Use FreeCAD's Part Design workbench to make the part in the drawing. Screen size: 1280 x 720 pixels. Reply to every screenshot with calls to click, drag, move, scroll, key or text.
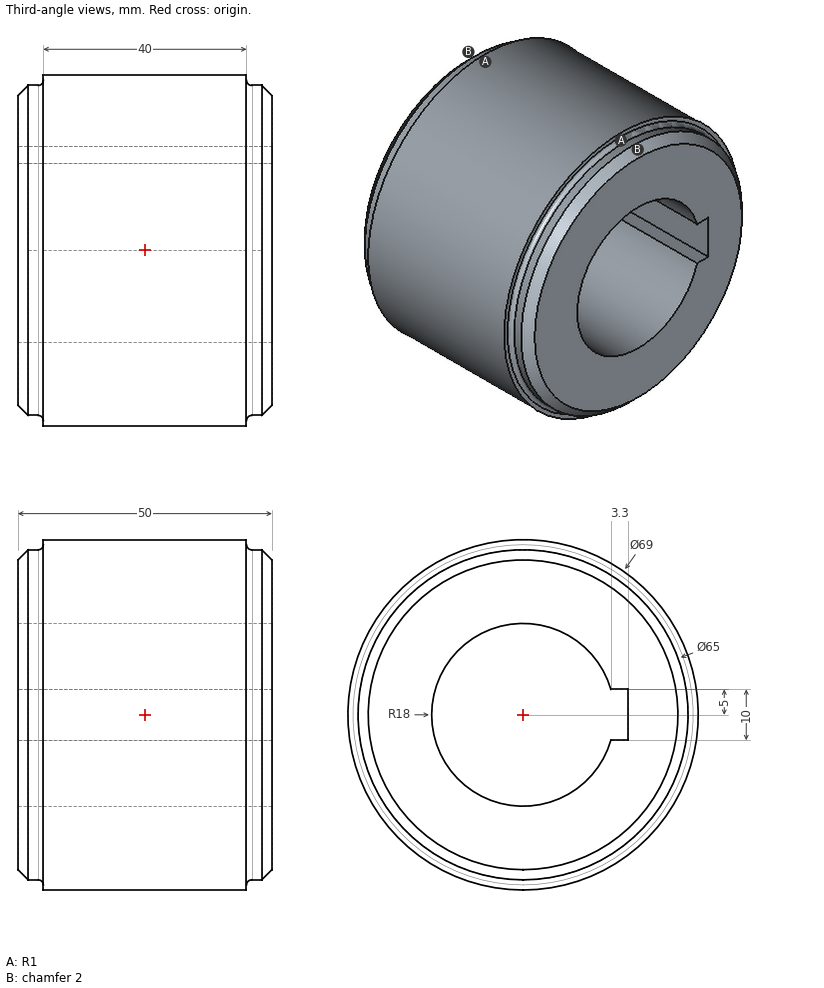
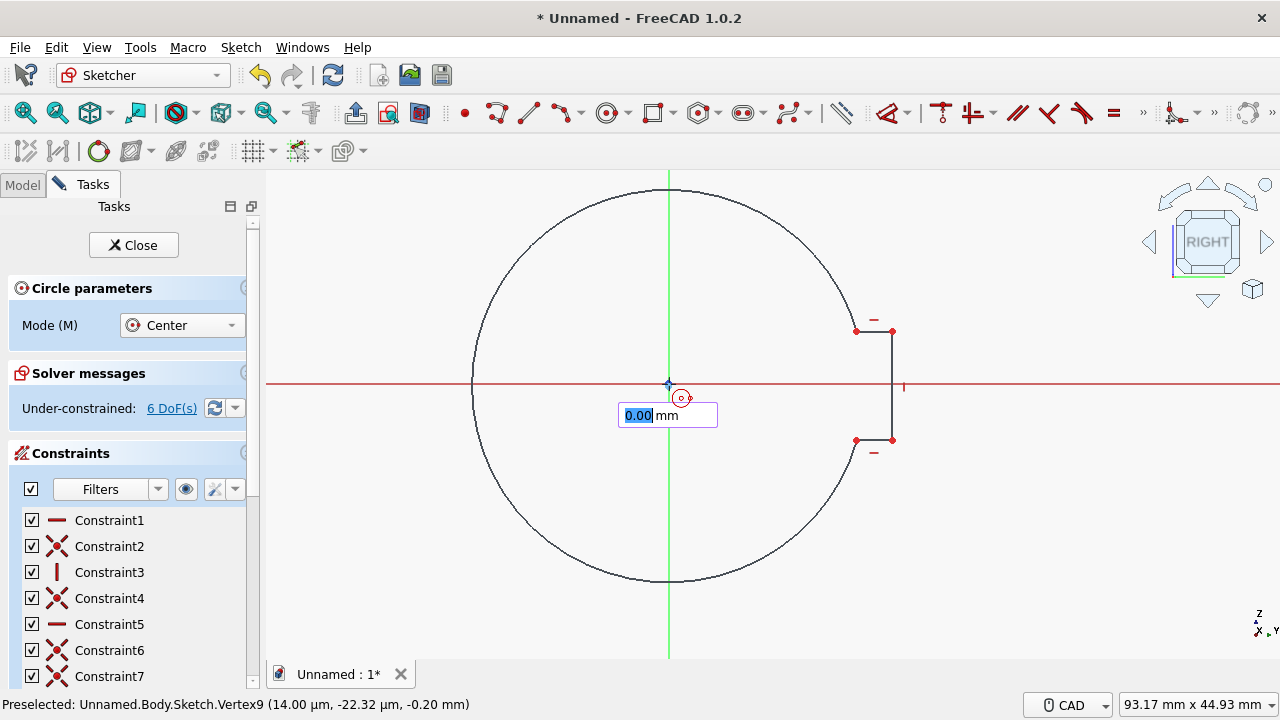
scroll(734, 439, down, 4)
move(817, 302)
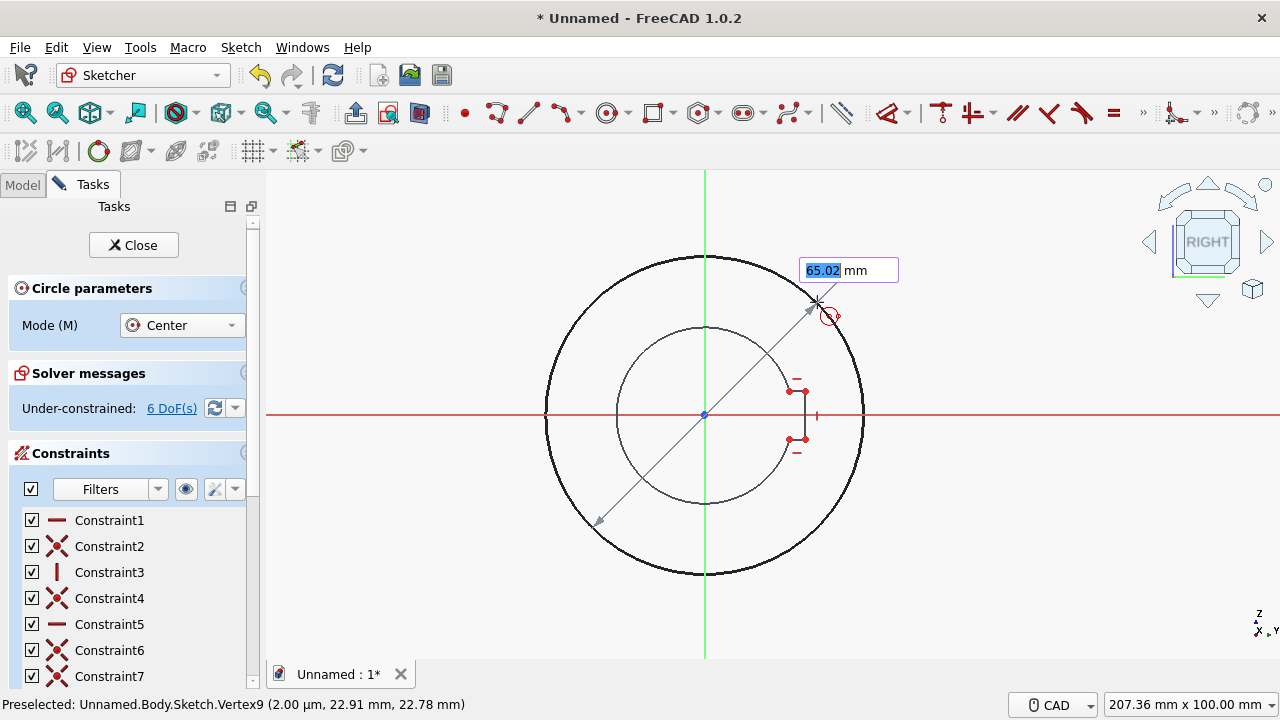
text(65)
key(Return)
key(Escape)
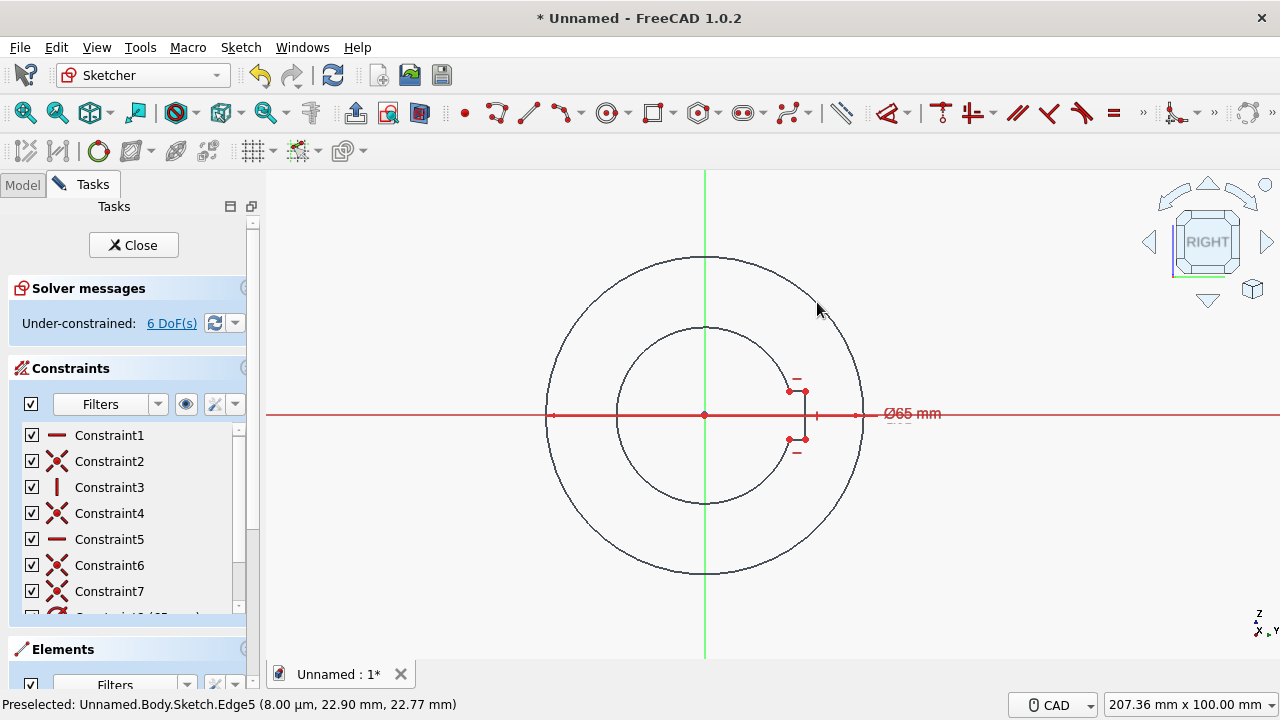
drag(695, 405, 715, 426)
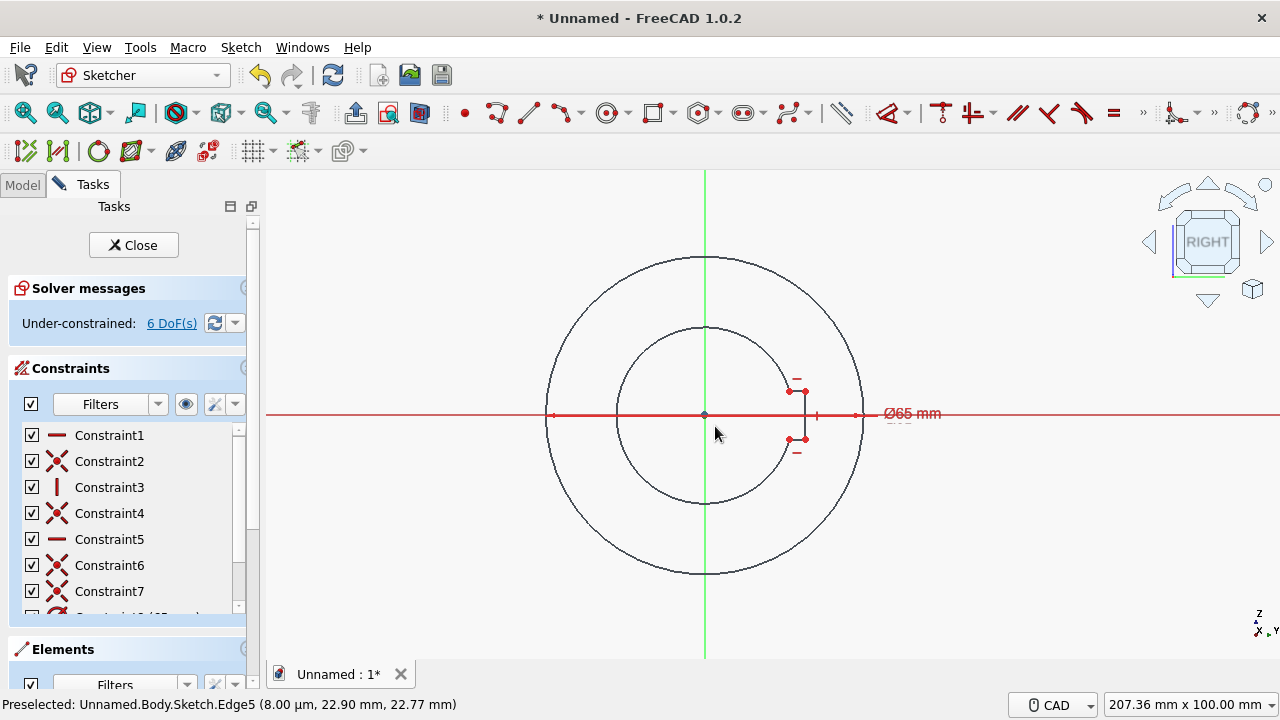
key(c)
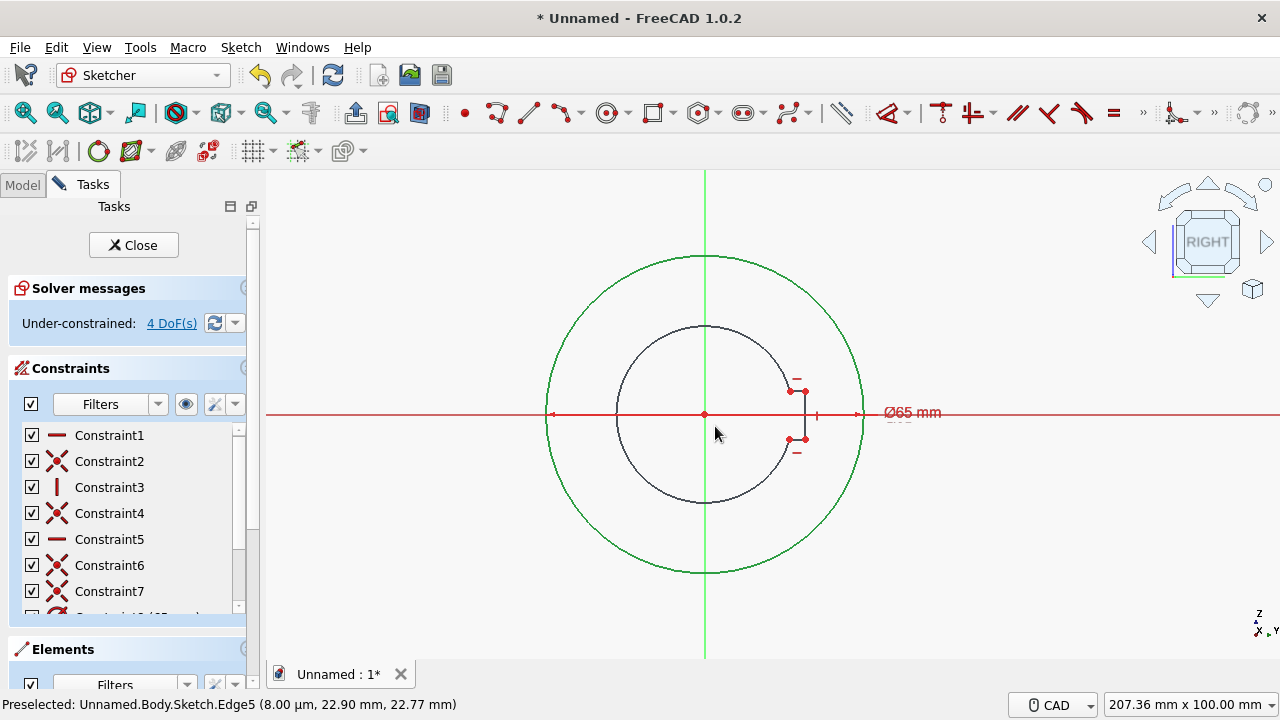
click(669, 334)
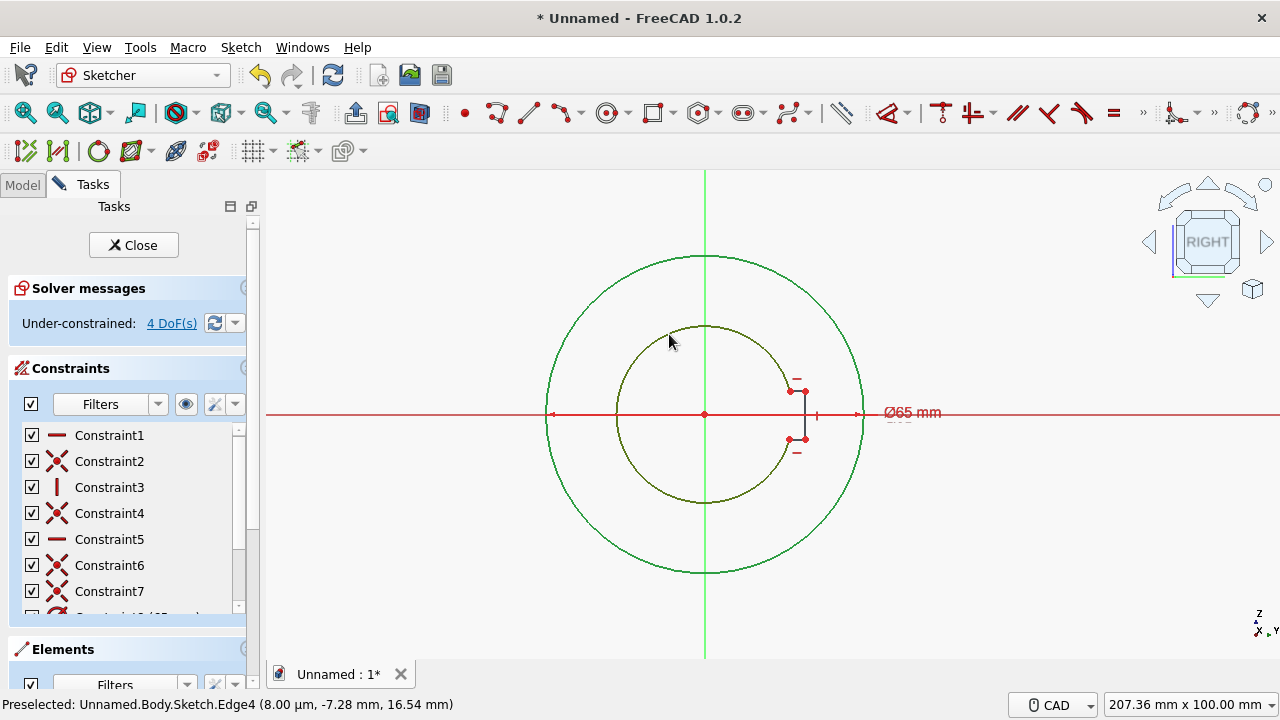
key(k)
key(r)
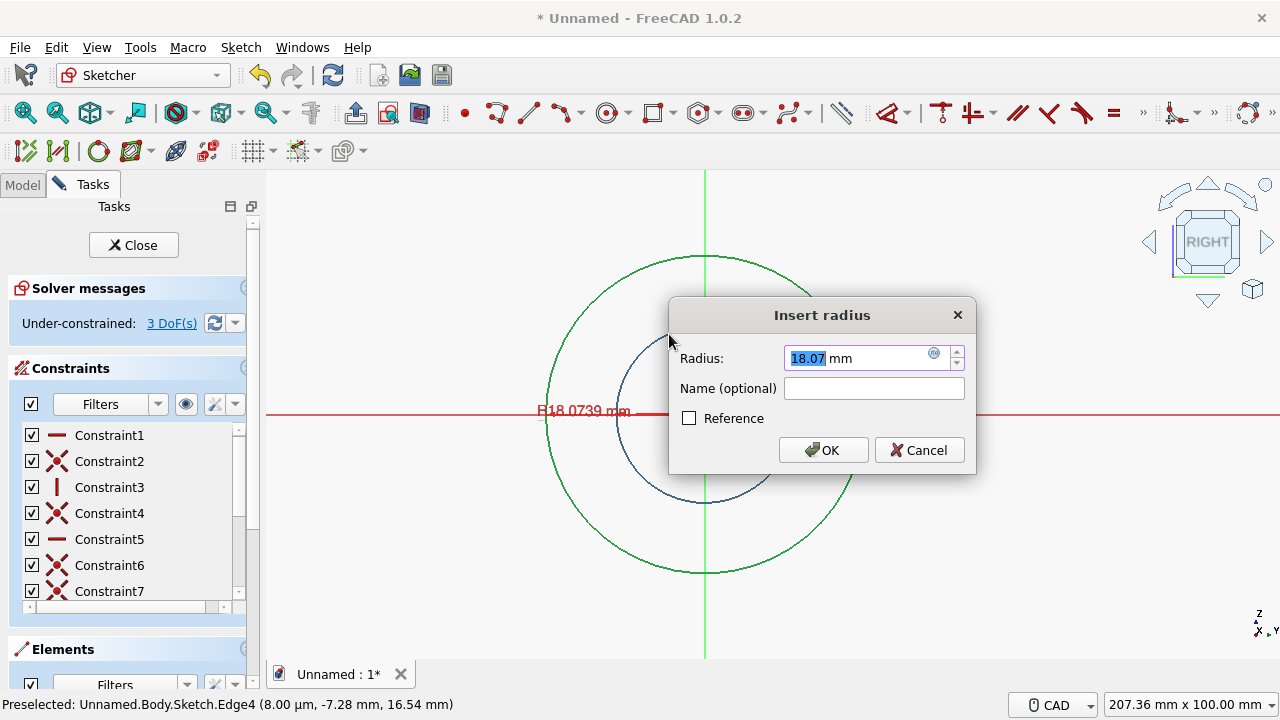
text(18)
key(Return)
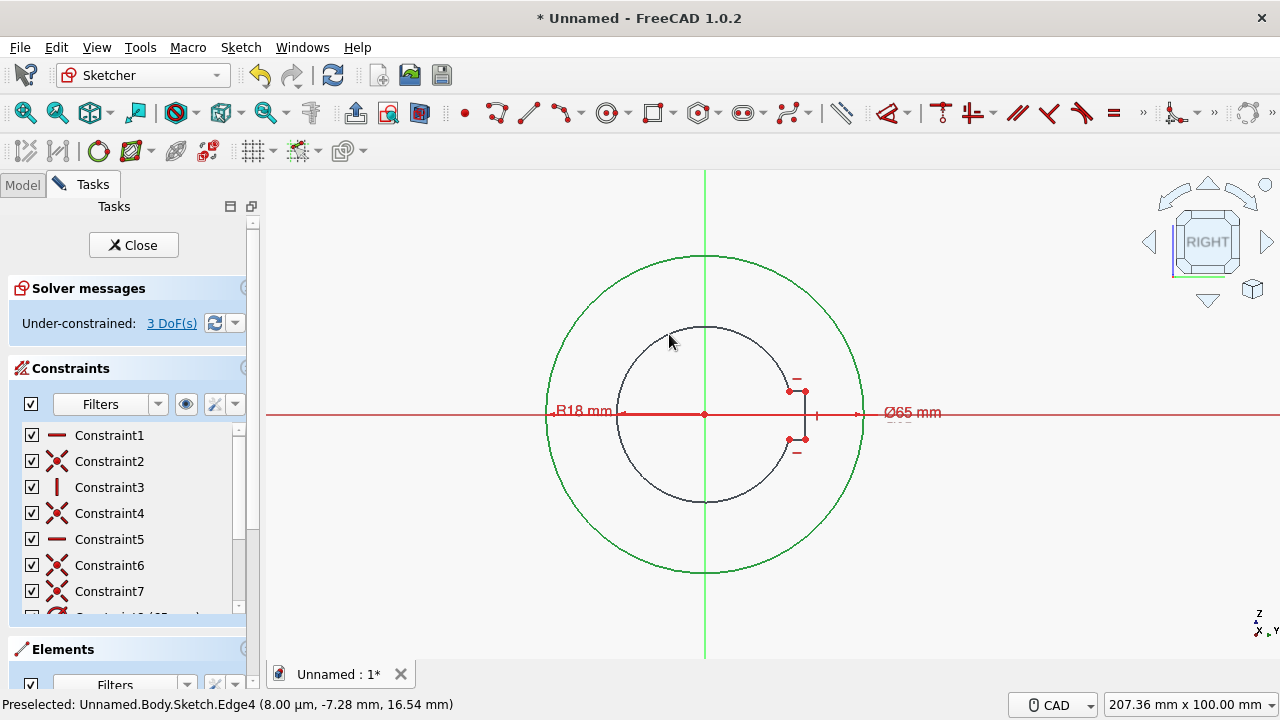
scroll(805, 425, up, 2)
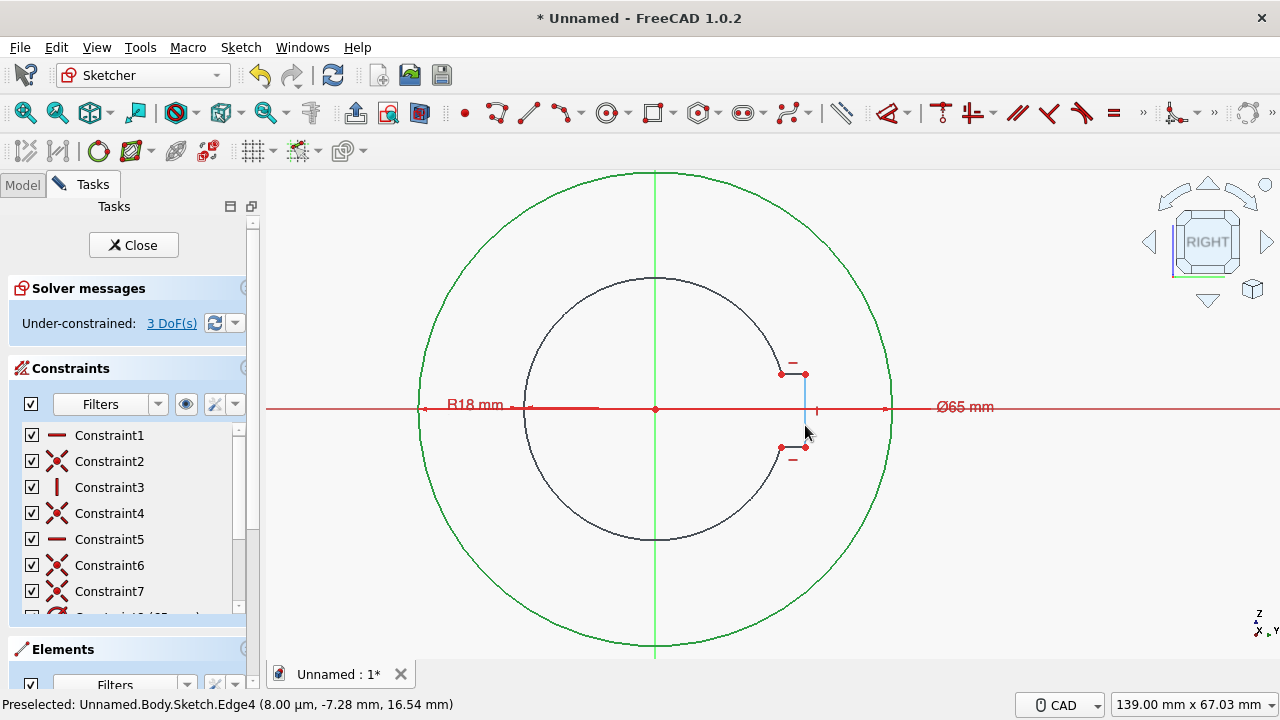
click(805, 425)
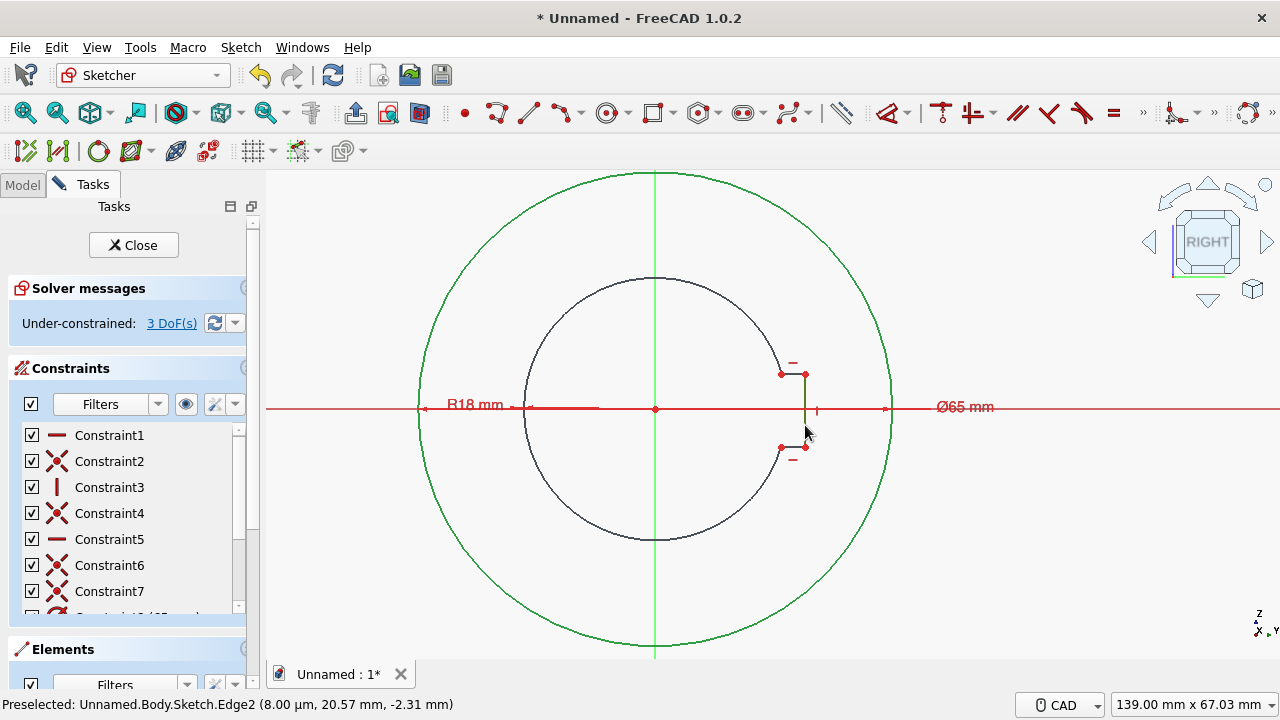
key(i)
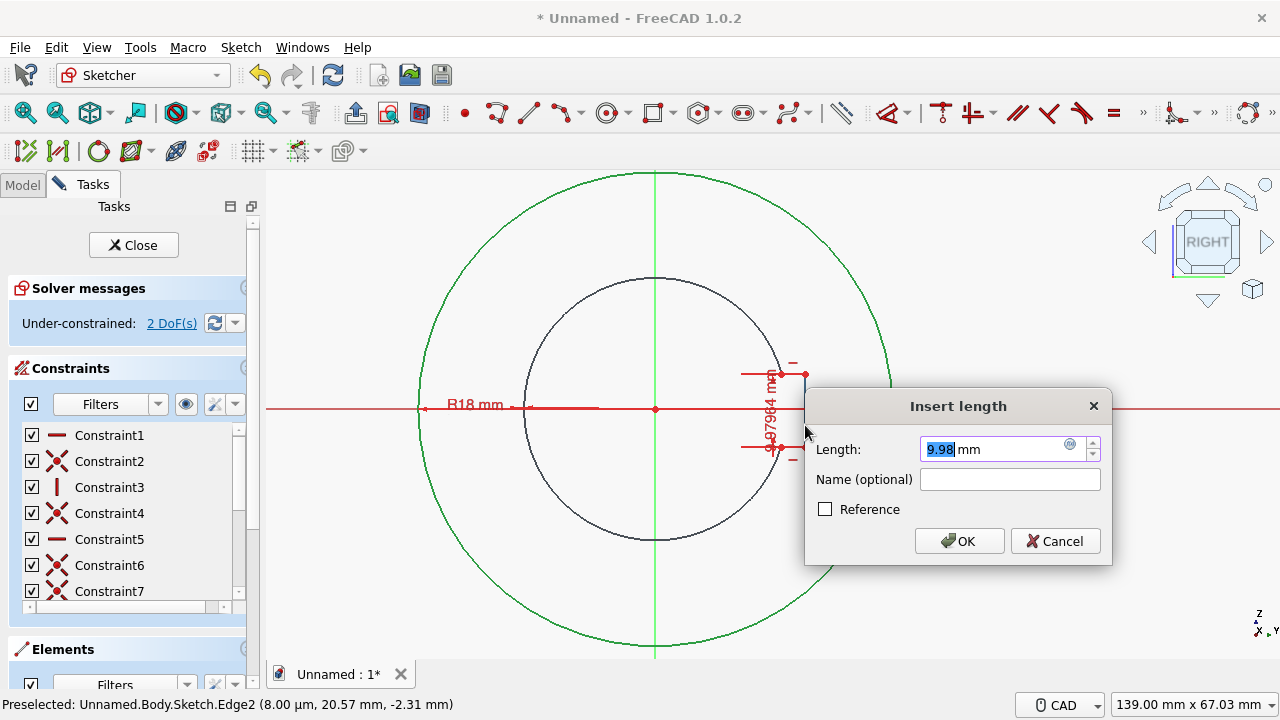
text(10)
key(Return)